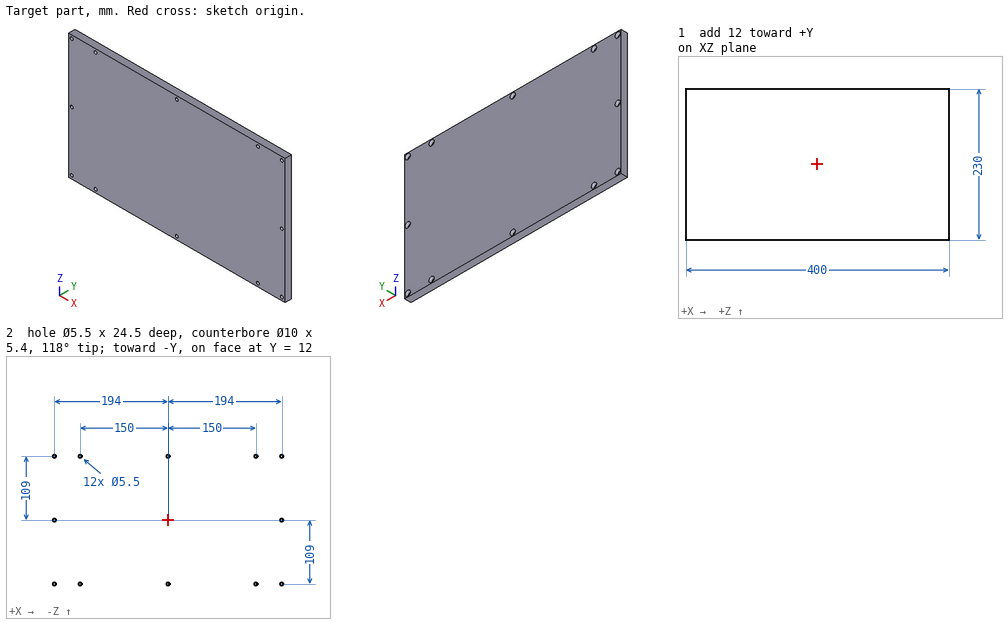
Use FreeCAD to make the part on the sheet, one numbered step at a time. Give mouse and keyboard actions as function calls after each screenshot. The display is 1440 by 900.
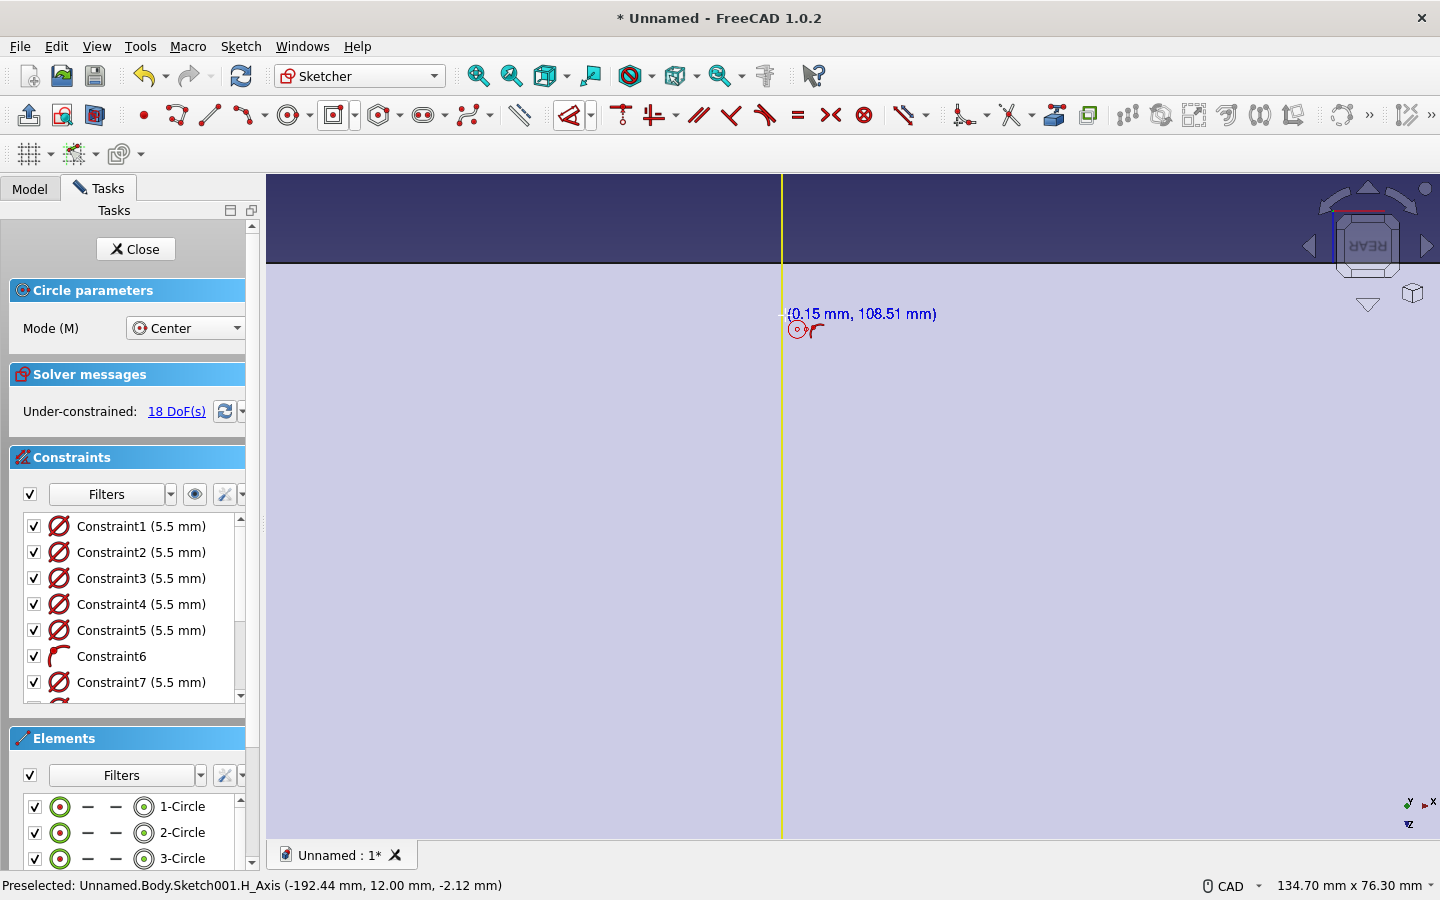
scroll(785, 315, down, 8)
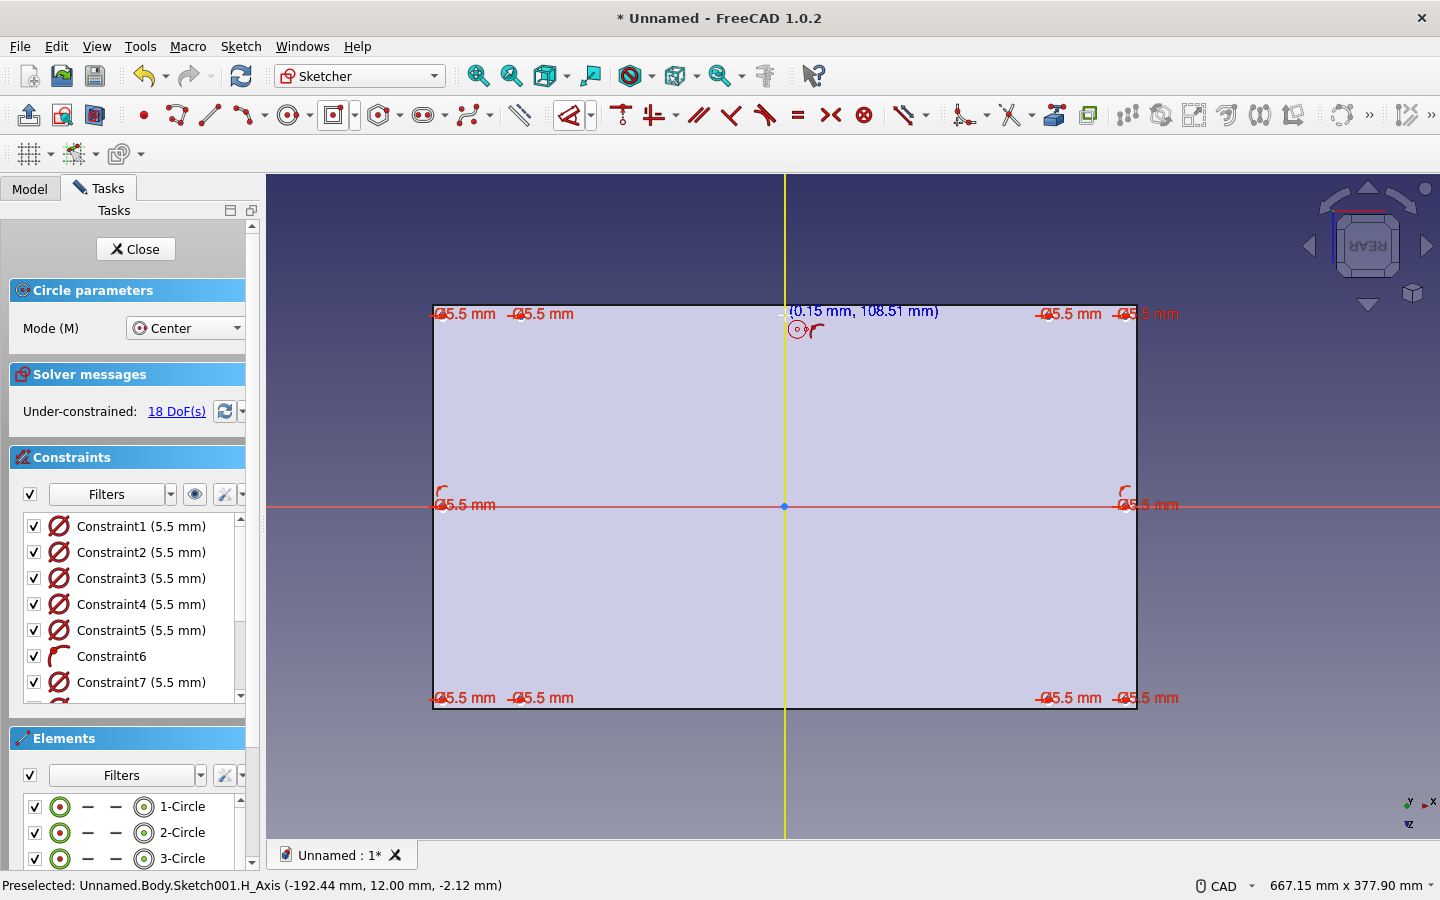
click(785, 315)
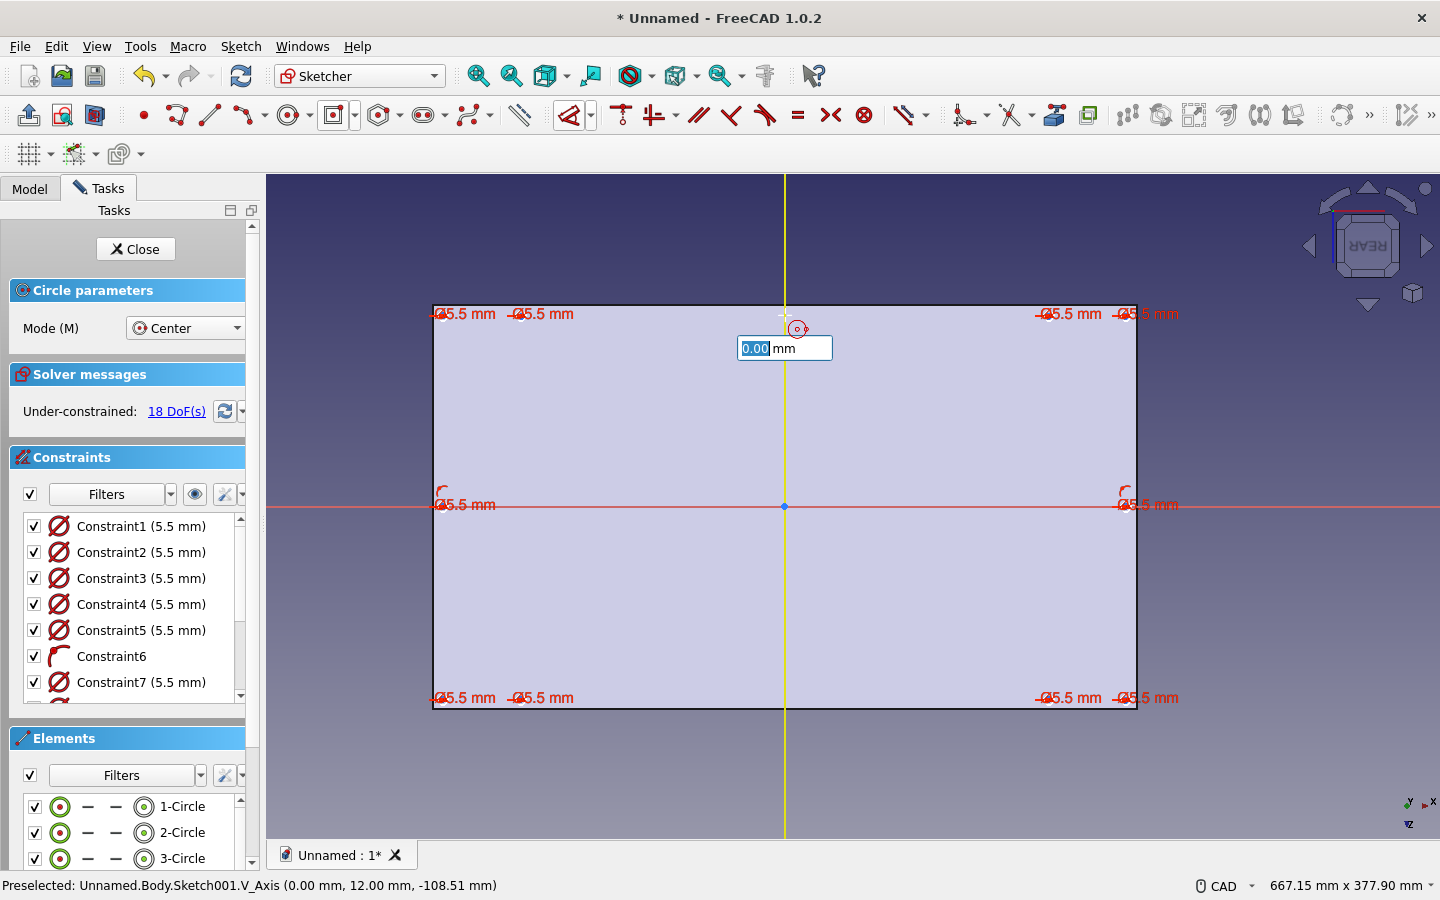
scroll(789, 313, up, 7)
move(789, 314)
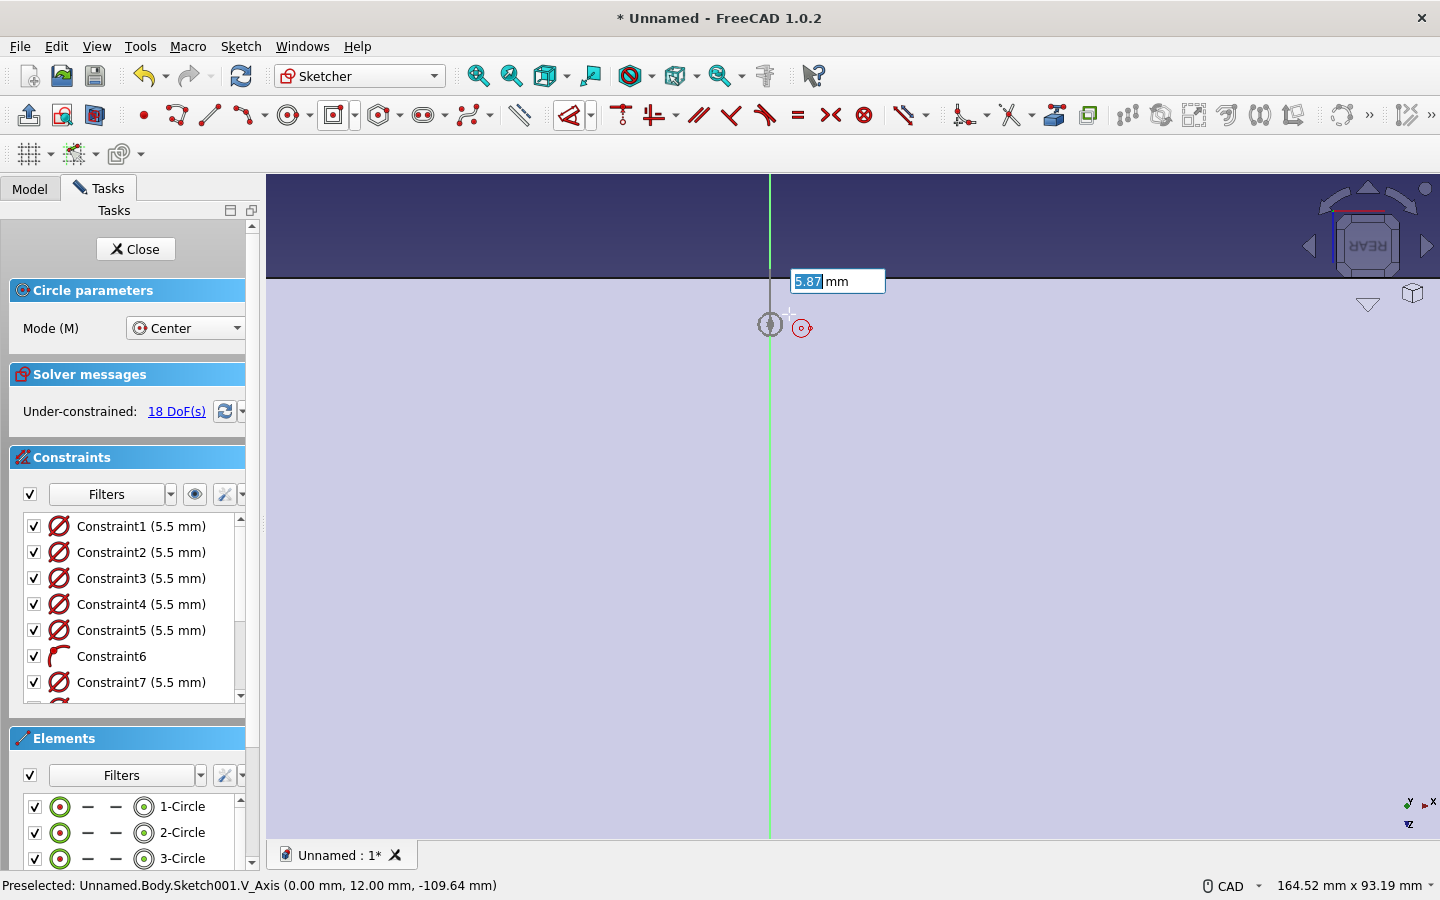
text(5.5)
key(Return)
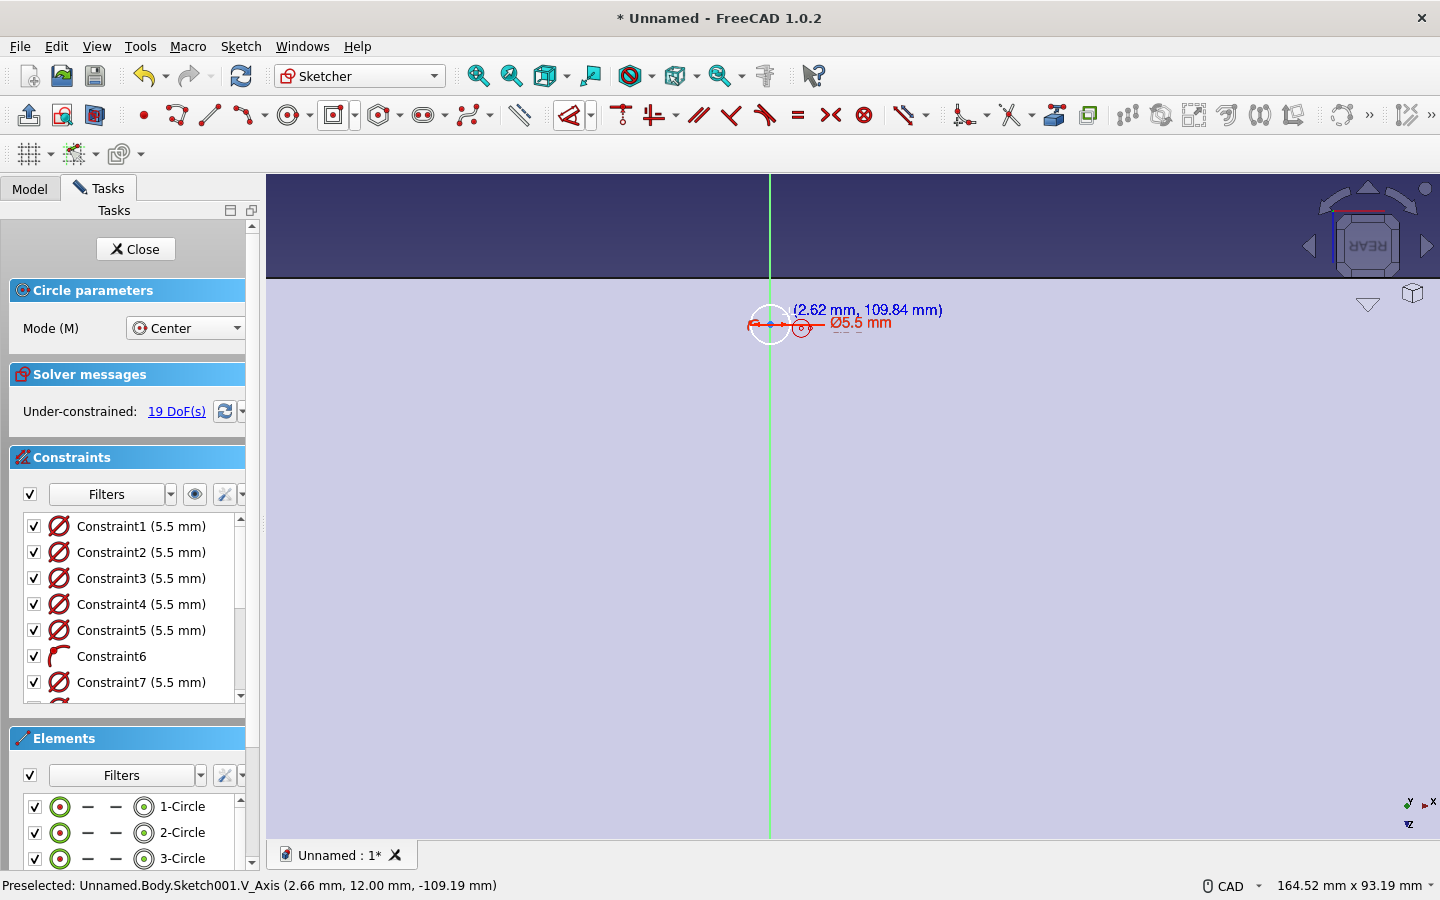
scroll(789, 313, down, 7)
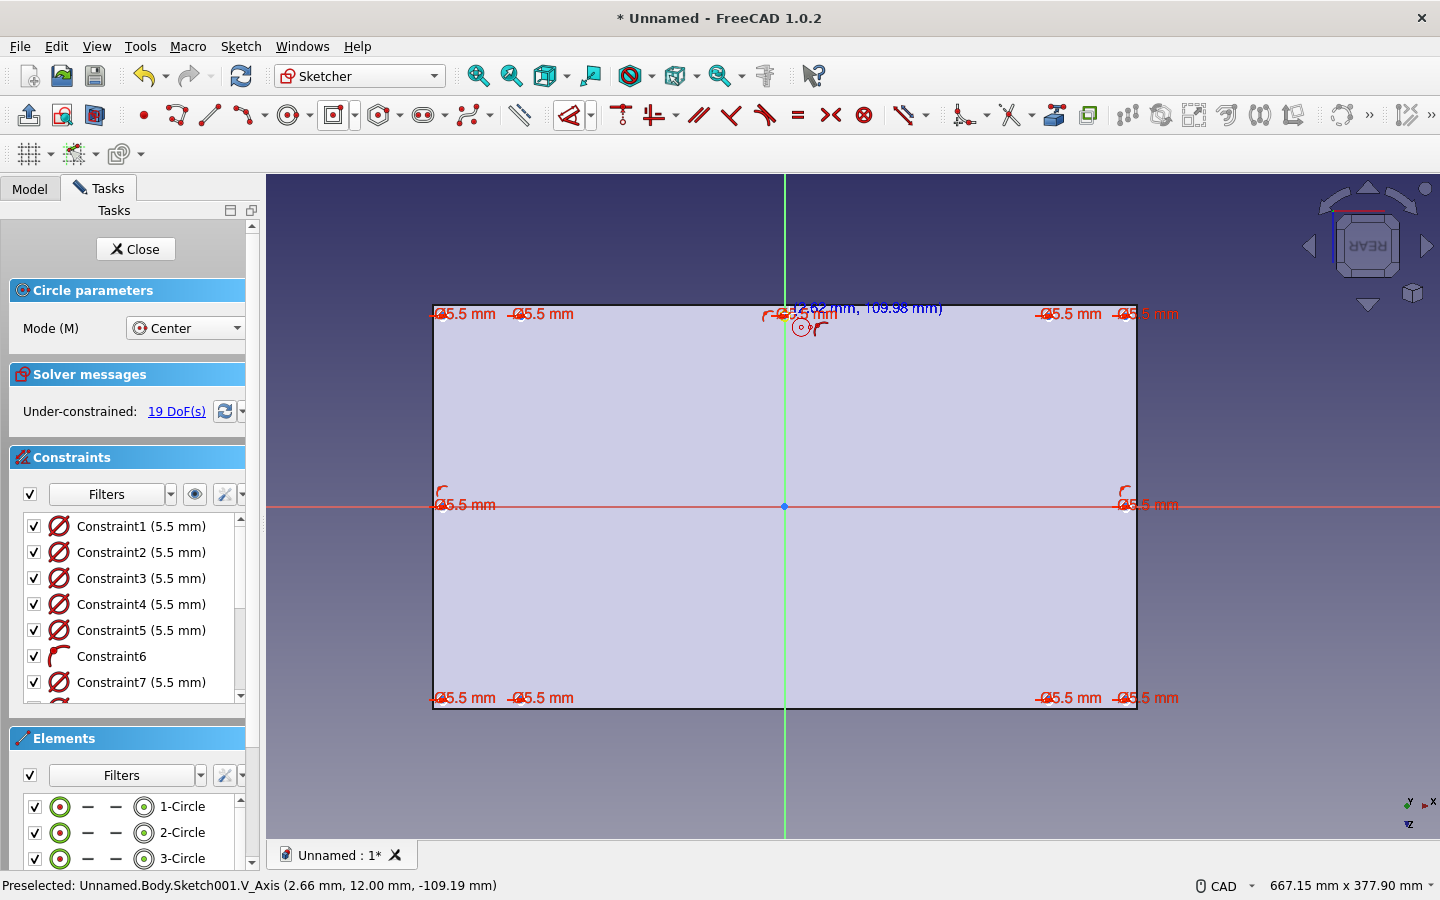
scroll(785, 699, up, 8)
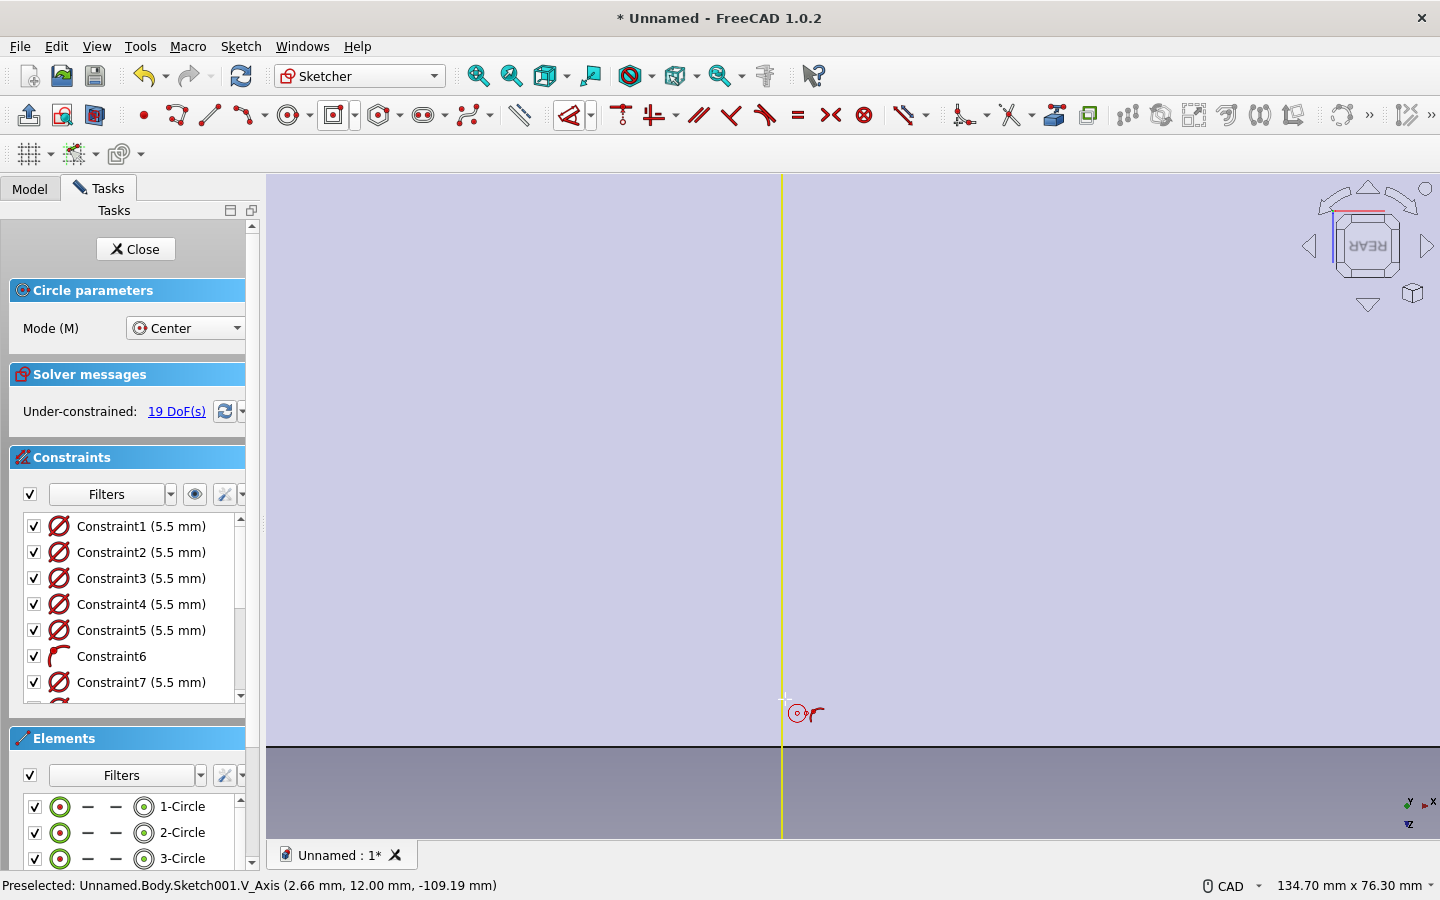
scroll(785, 699, down, 8)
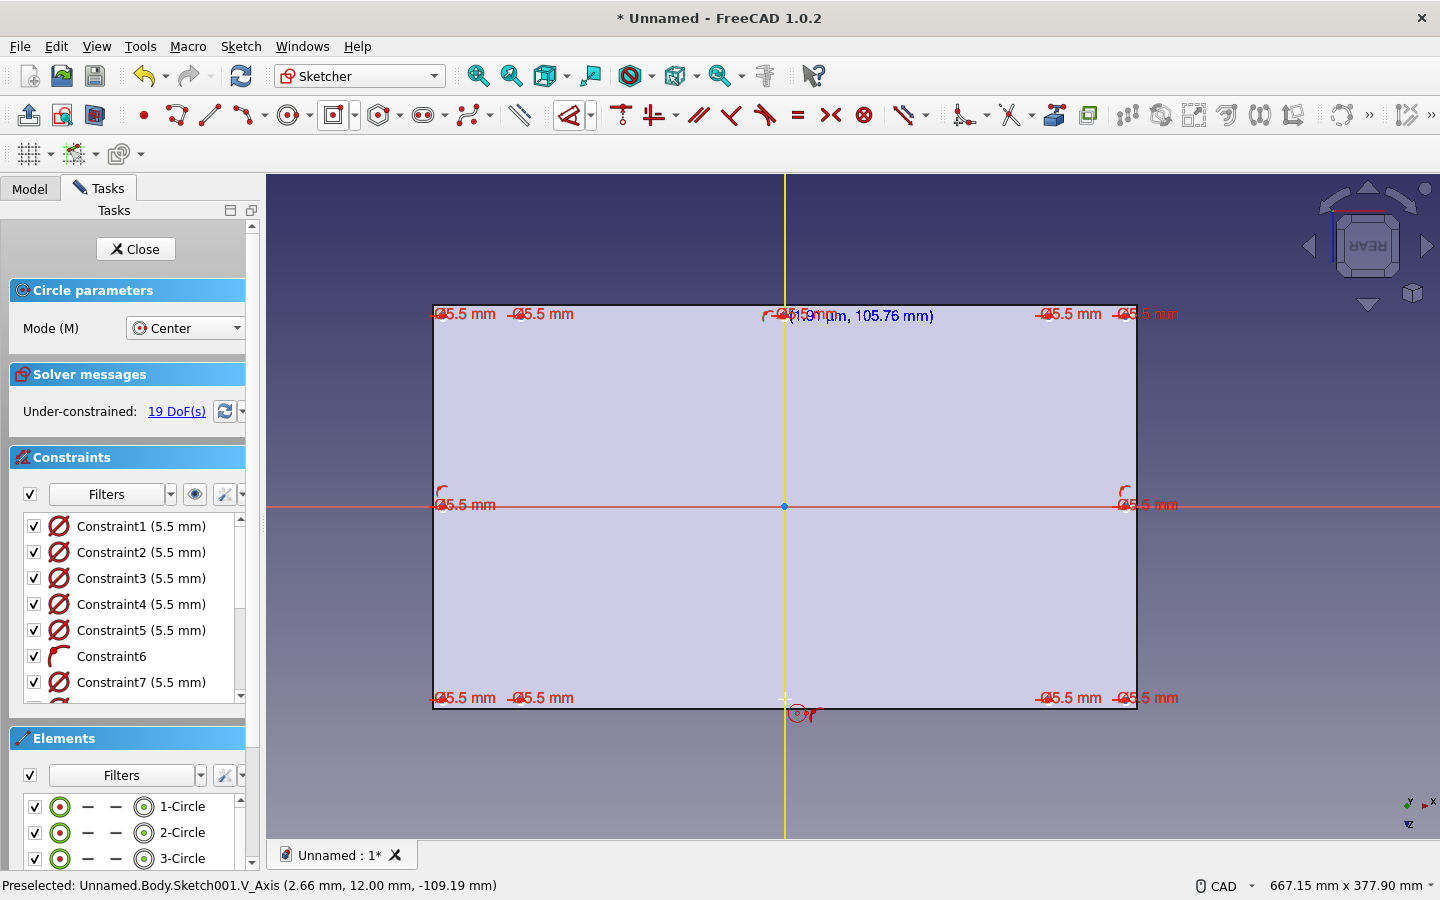
click(785, 699)